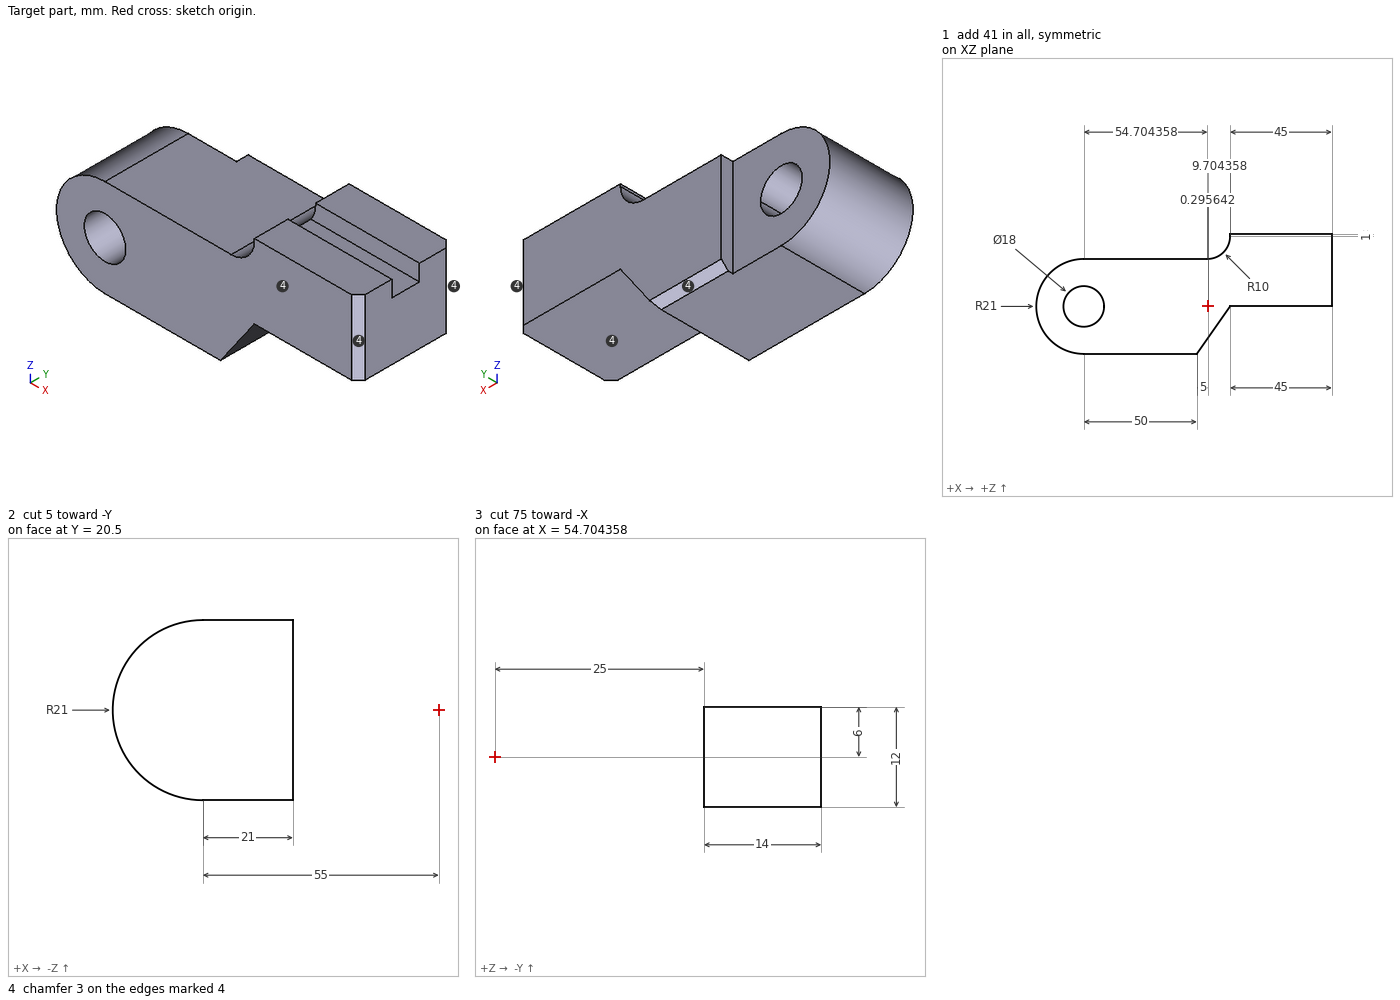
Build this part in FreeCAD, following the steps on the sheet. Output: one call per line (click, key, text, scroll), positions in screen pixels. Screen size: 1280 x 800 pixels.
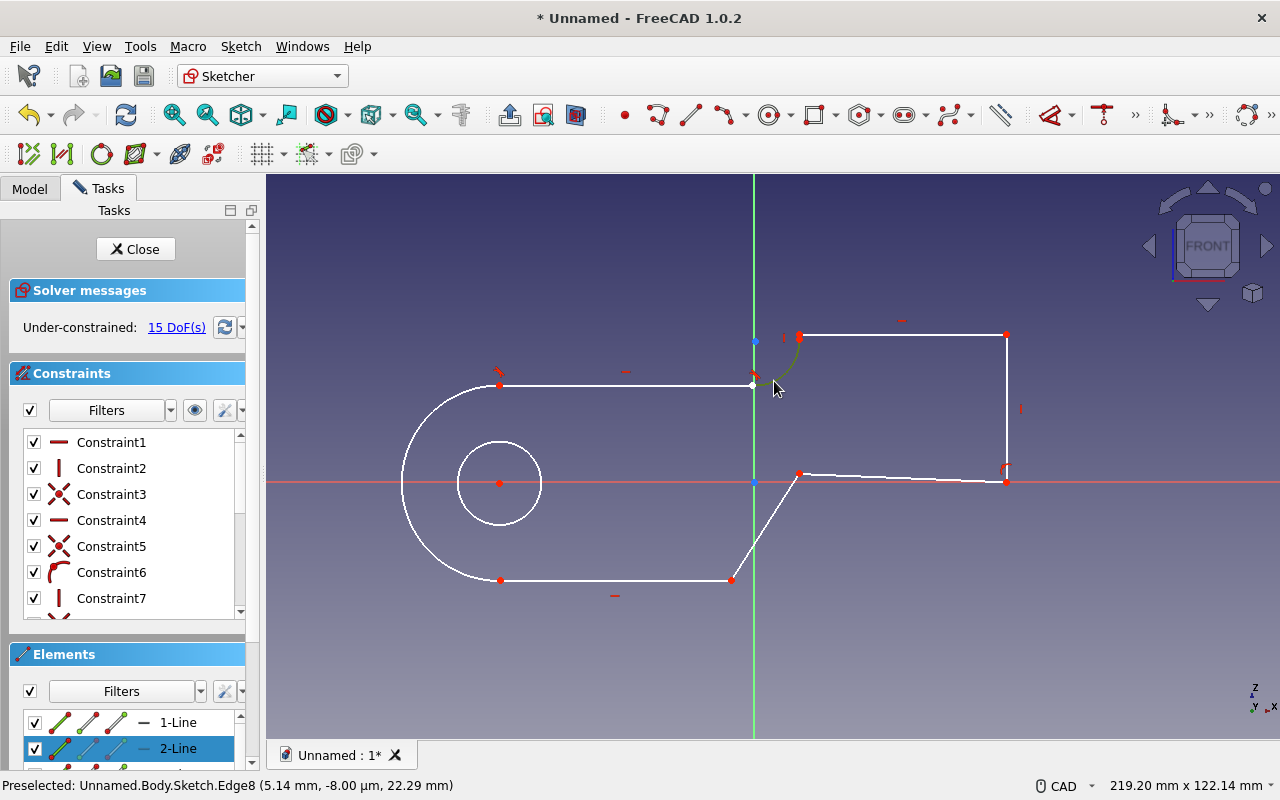
key(t)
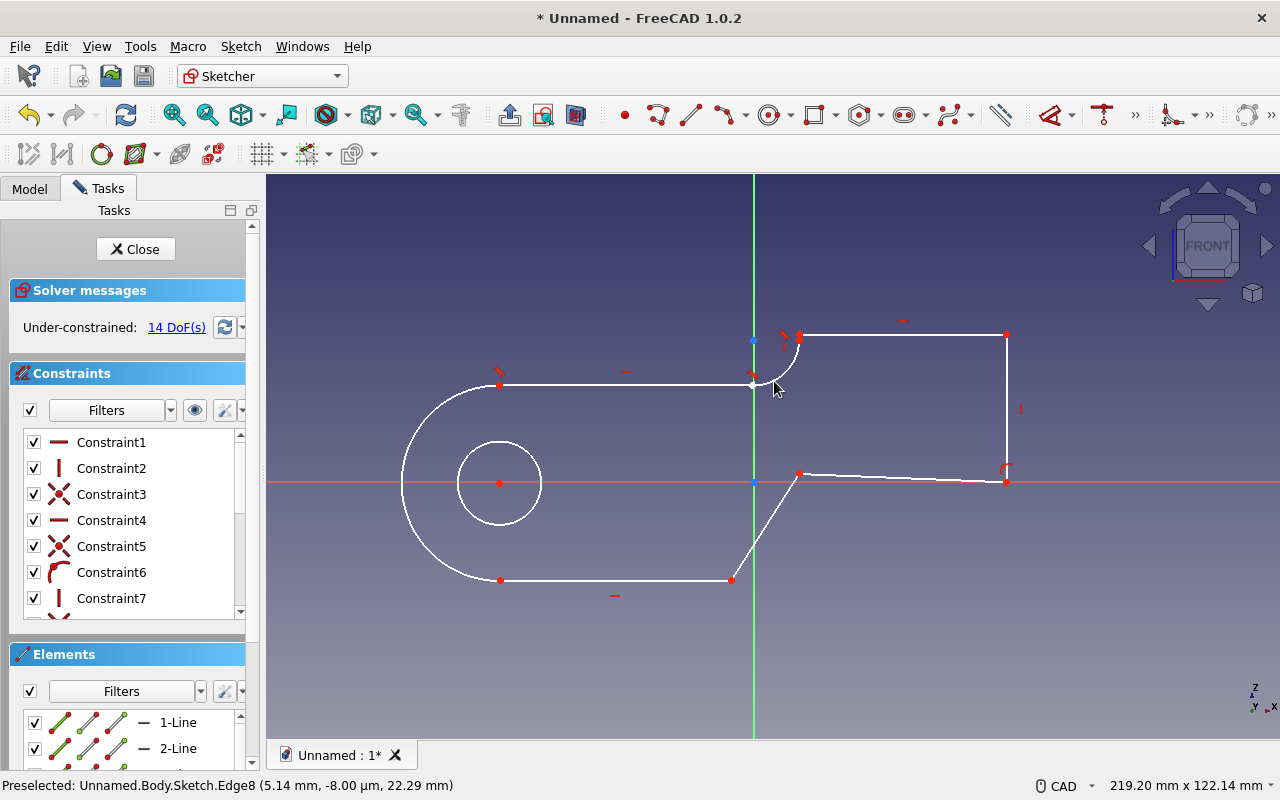
click(662, 581)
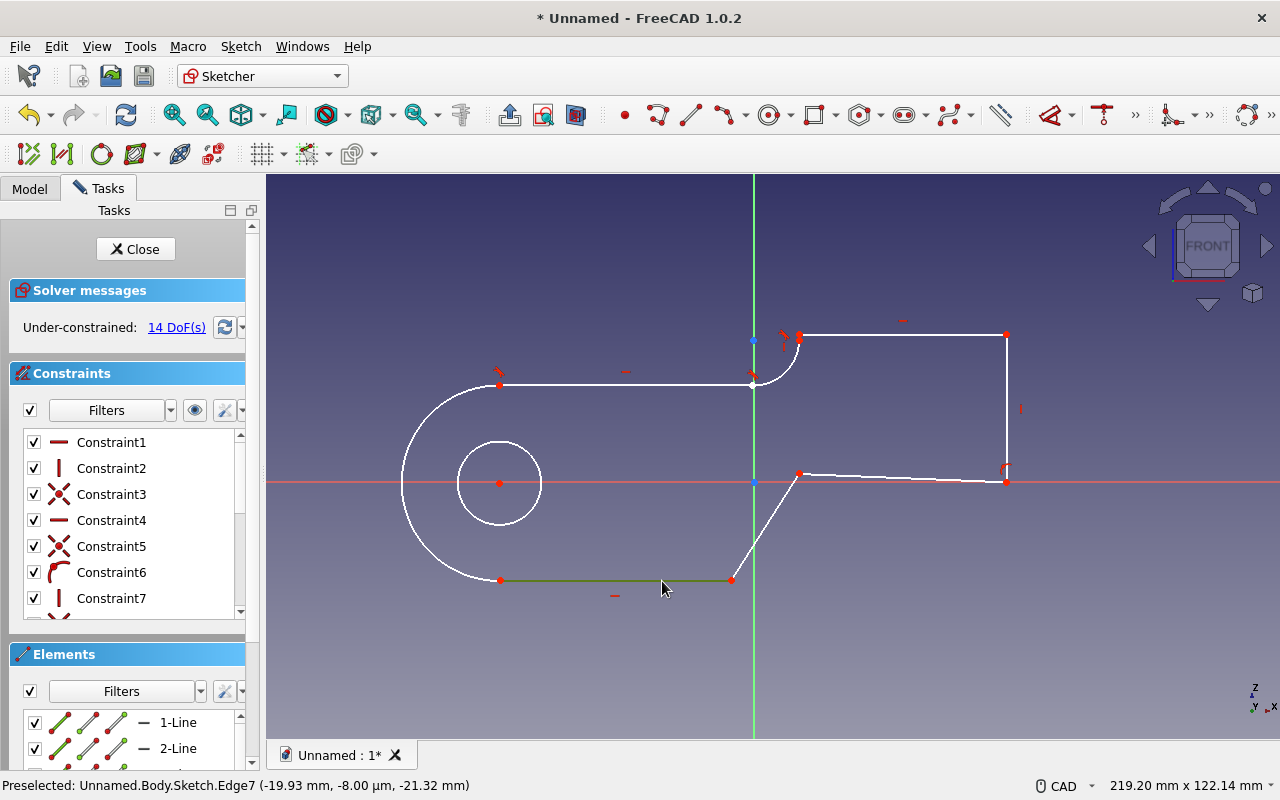
click(420, 426)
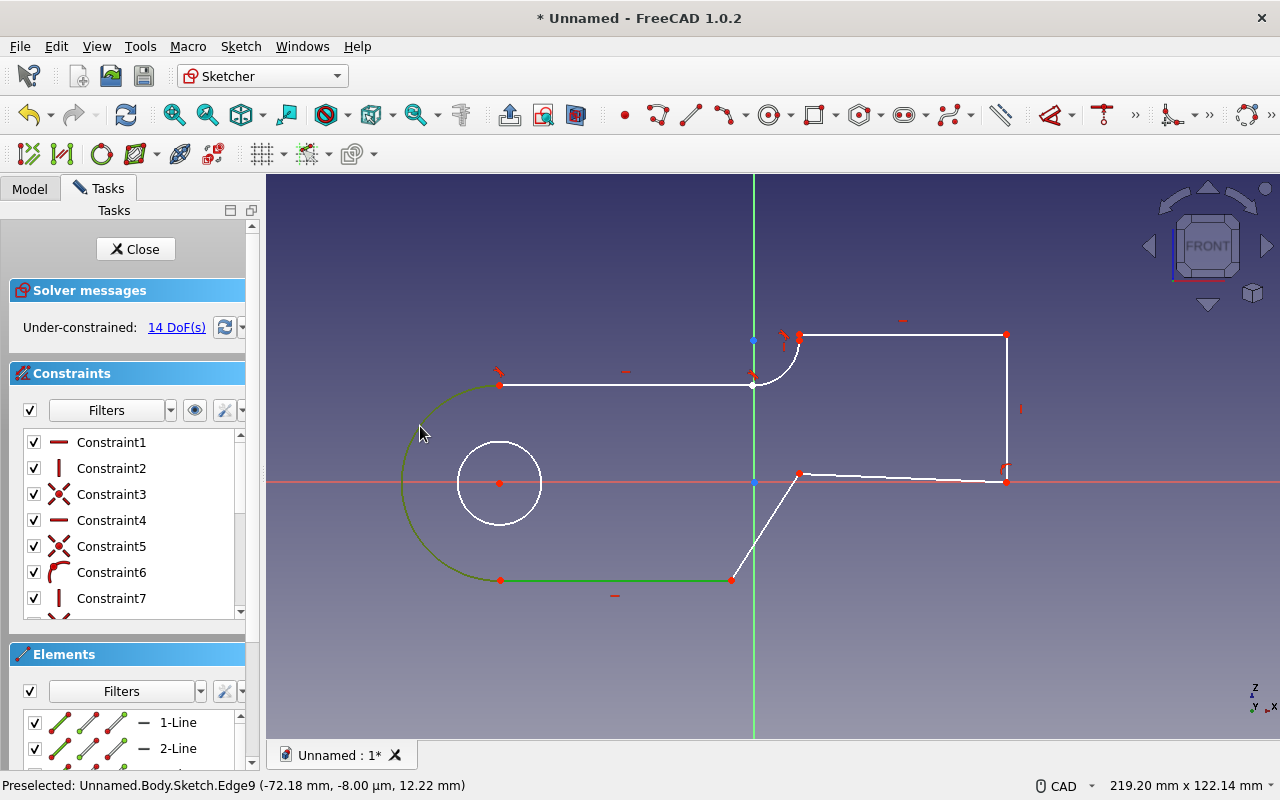
key(t)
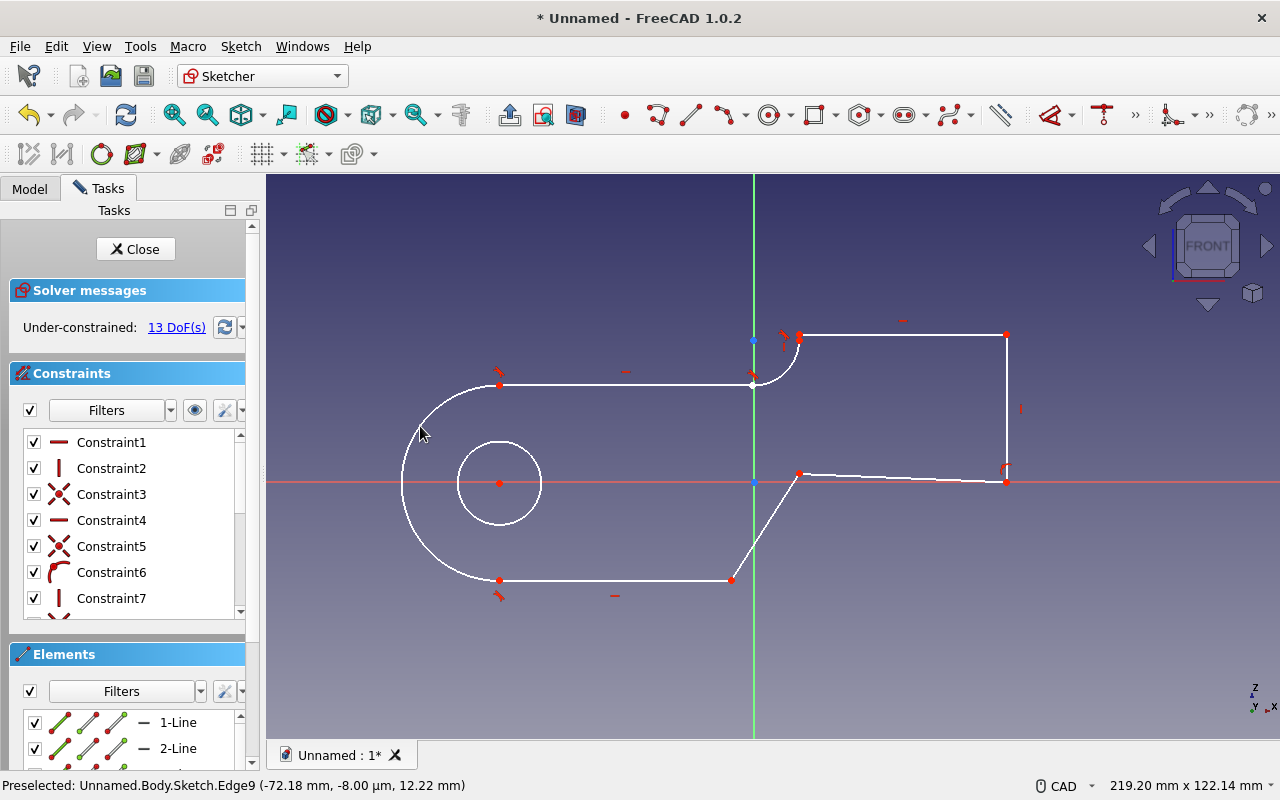
click(945, 480)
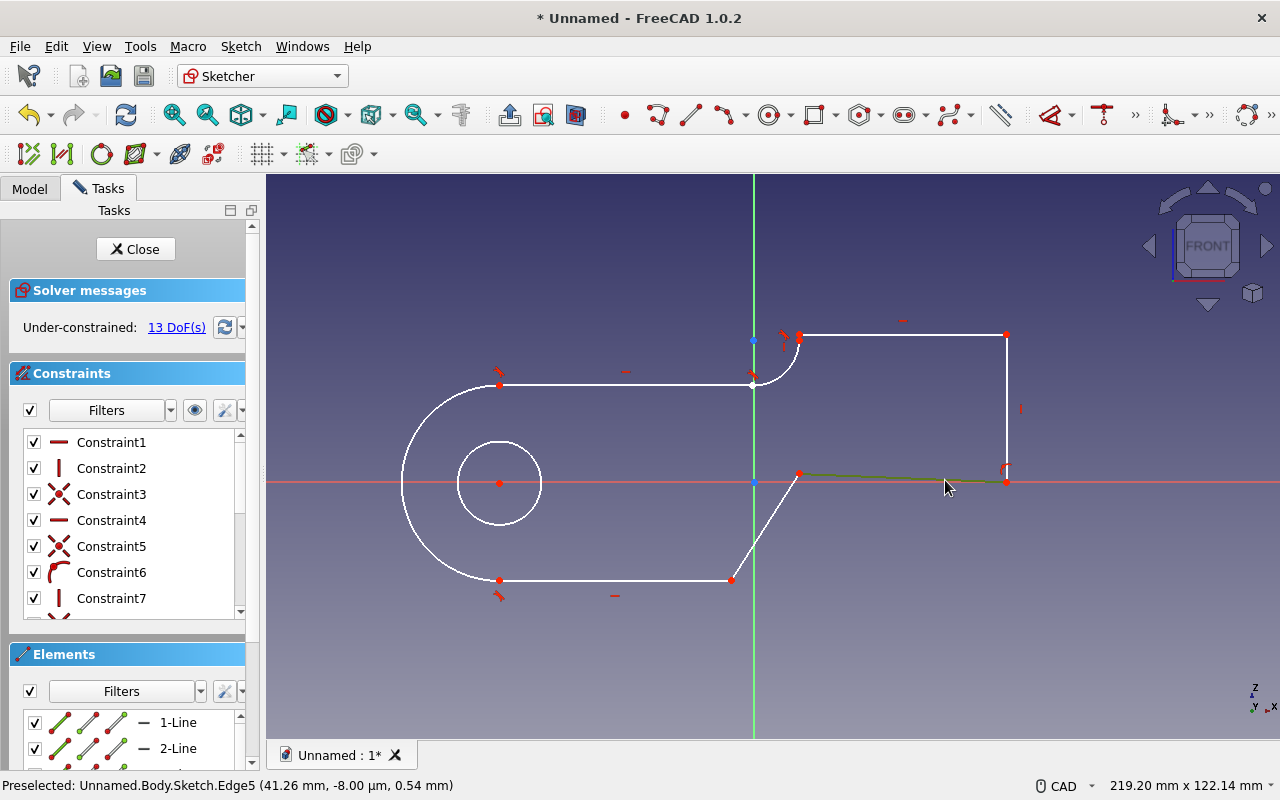
key(h)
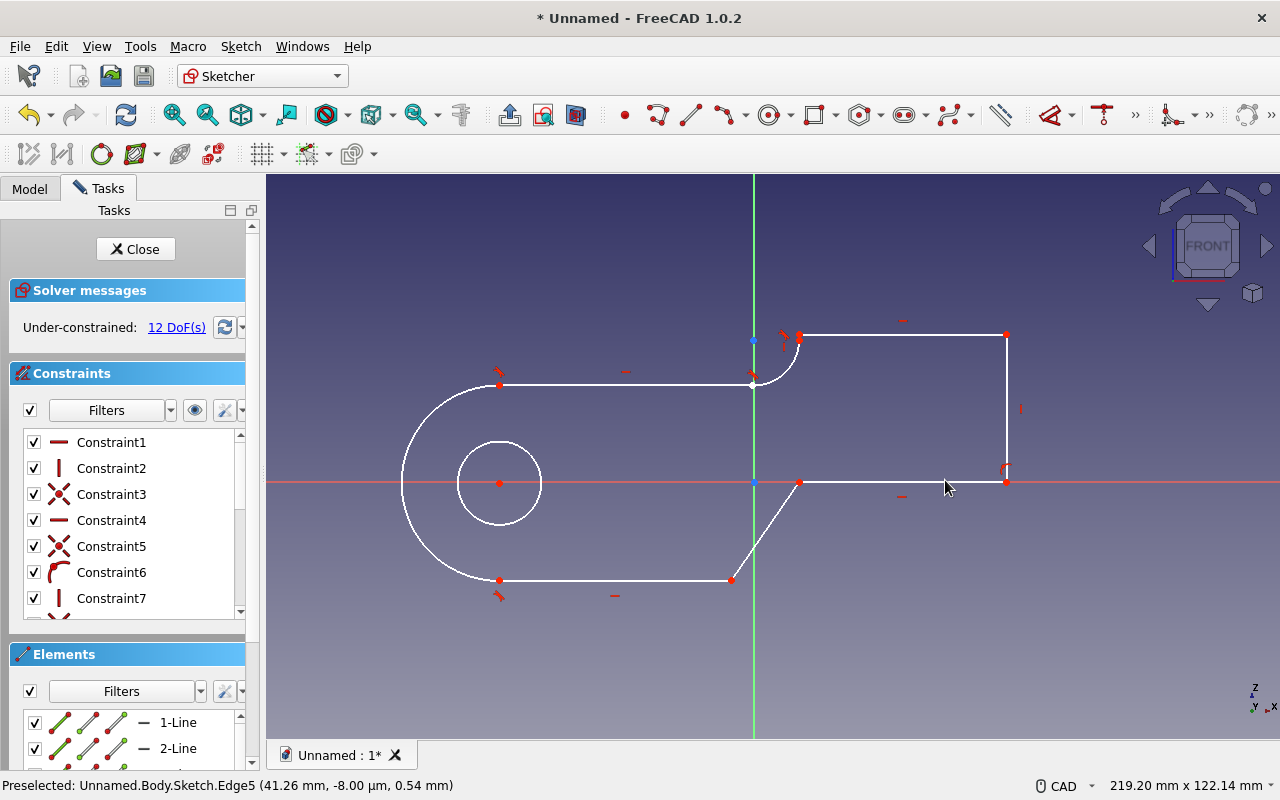
click(499, 483)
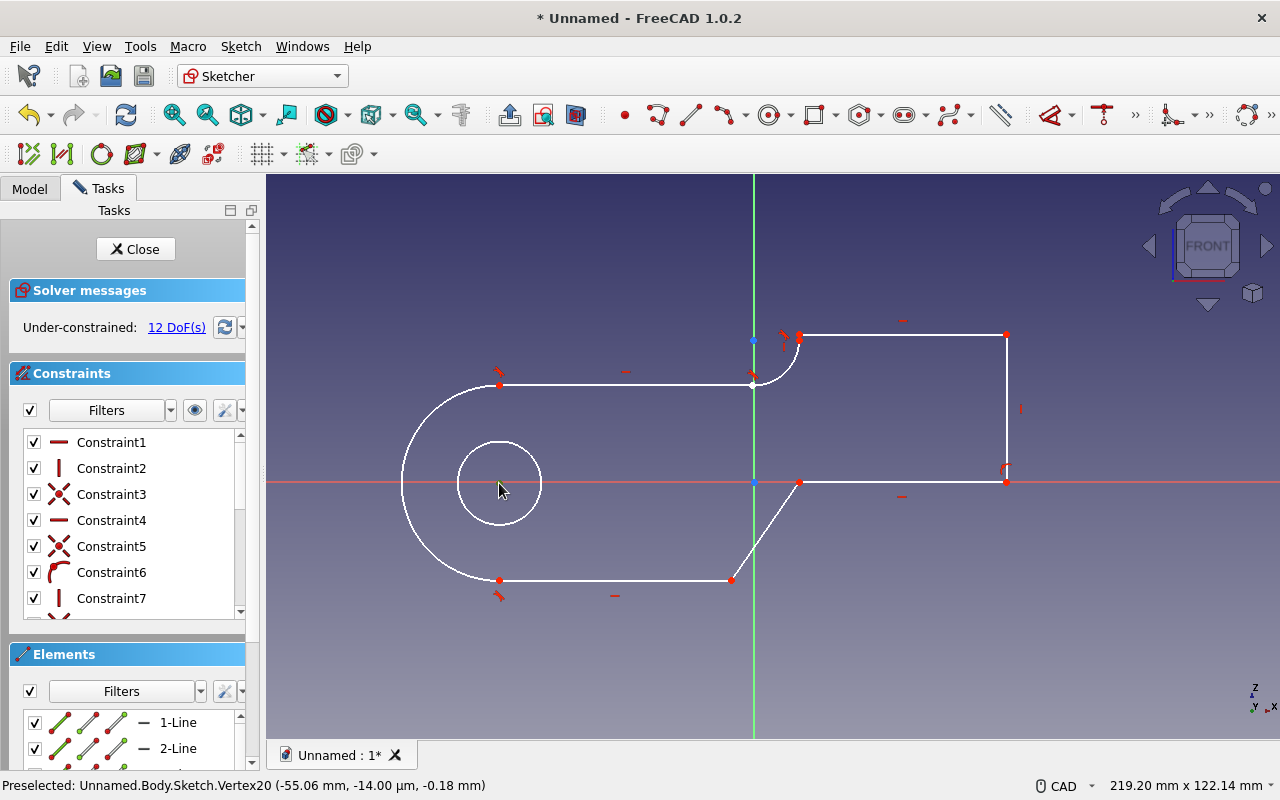
click(353, 482)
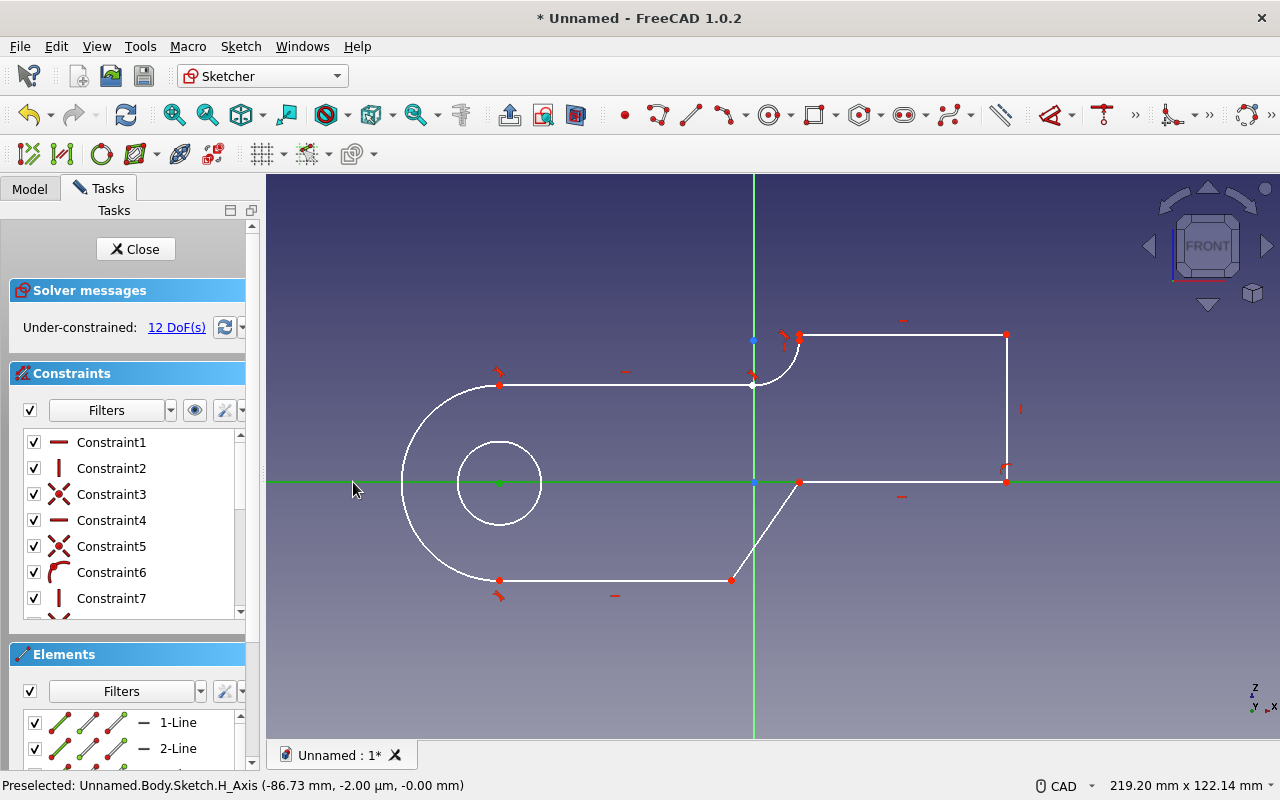
key(c)